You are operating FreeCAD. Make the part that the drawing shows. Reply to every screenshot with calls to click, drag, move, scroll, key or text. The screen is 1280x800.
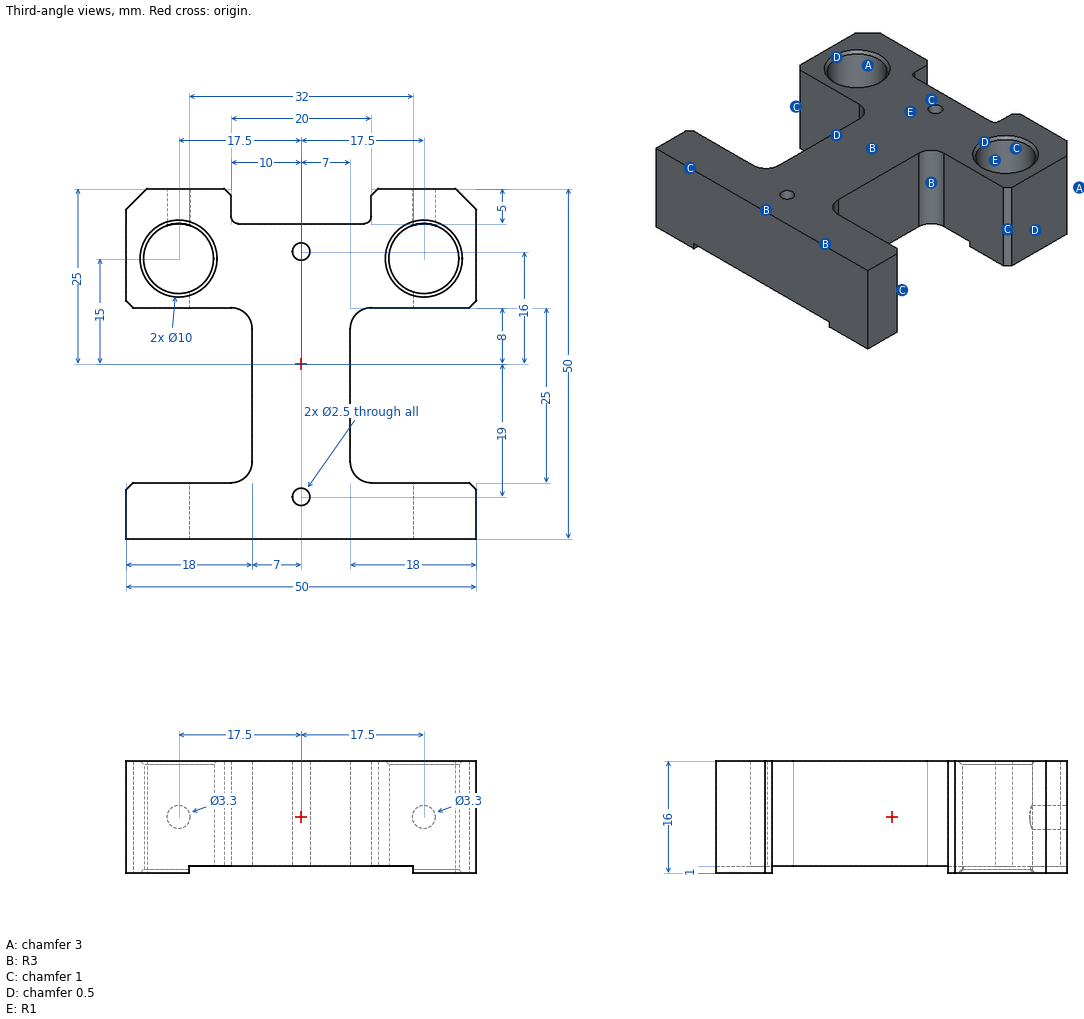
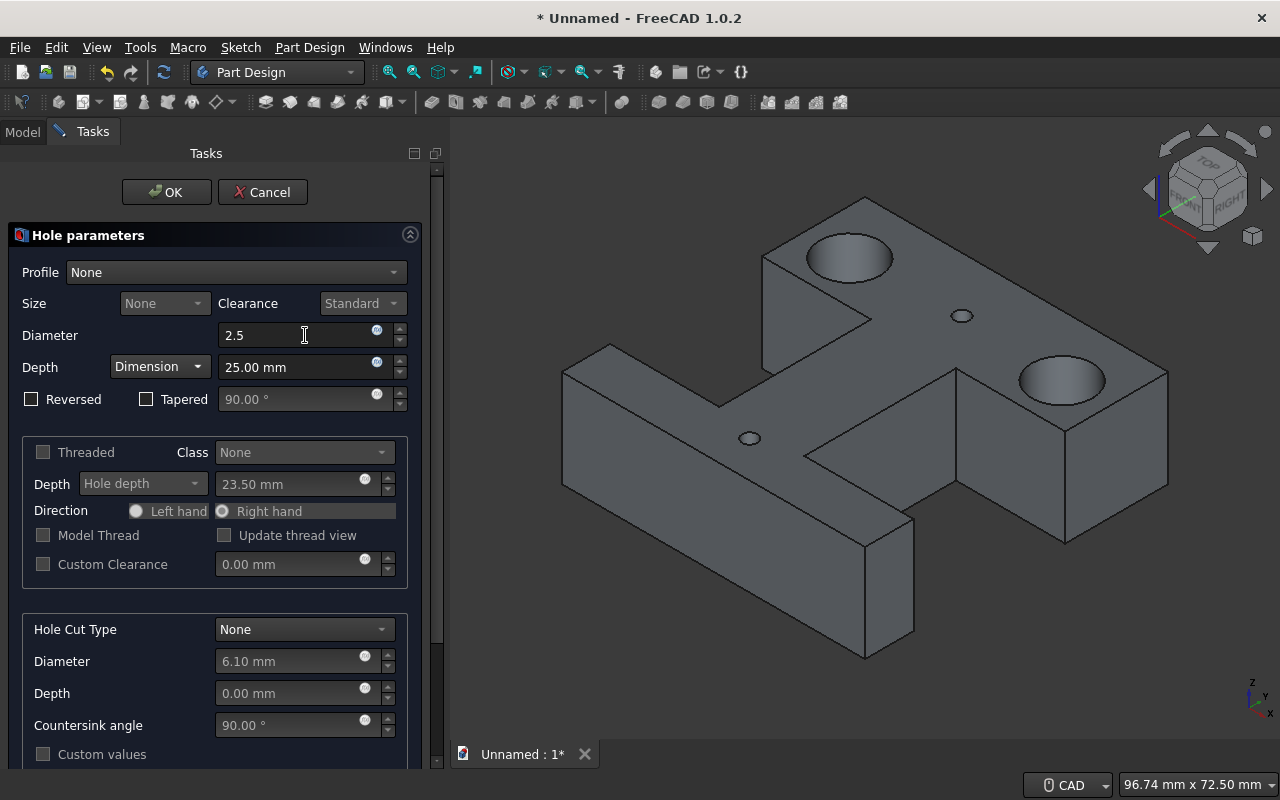
click(161, 366)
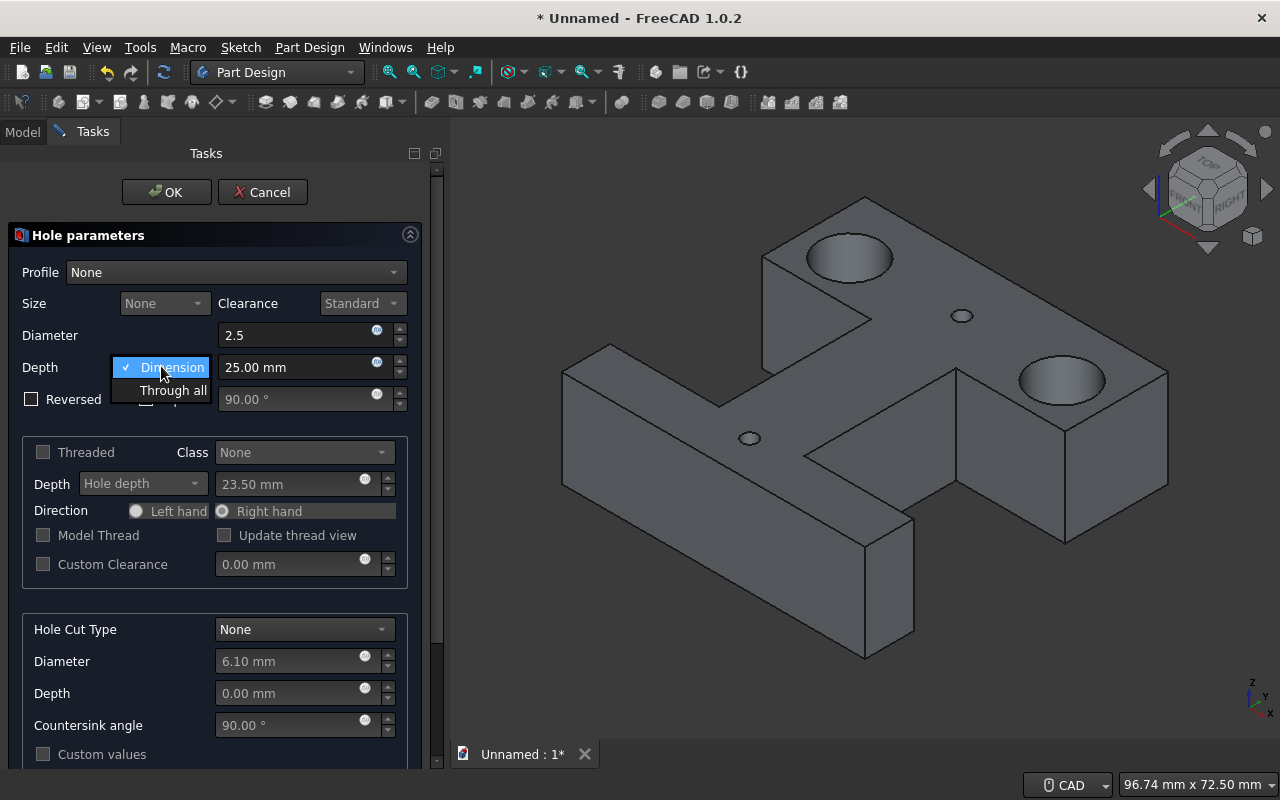
click(160, 390)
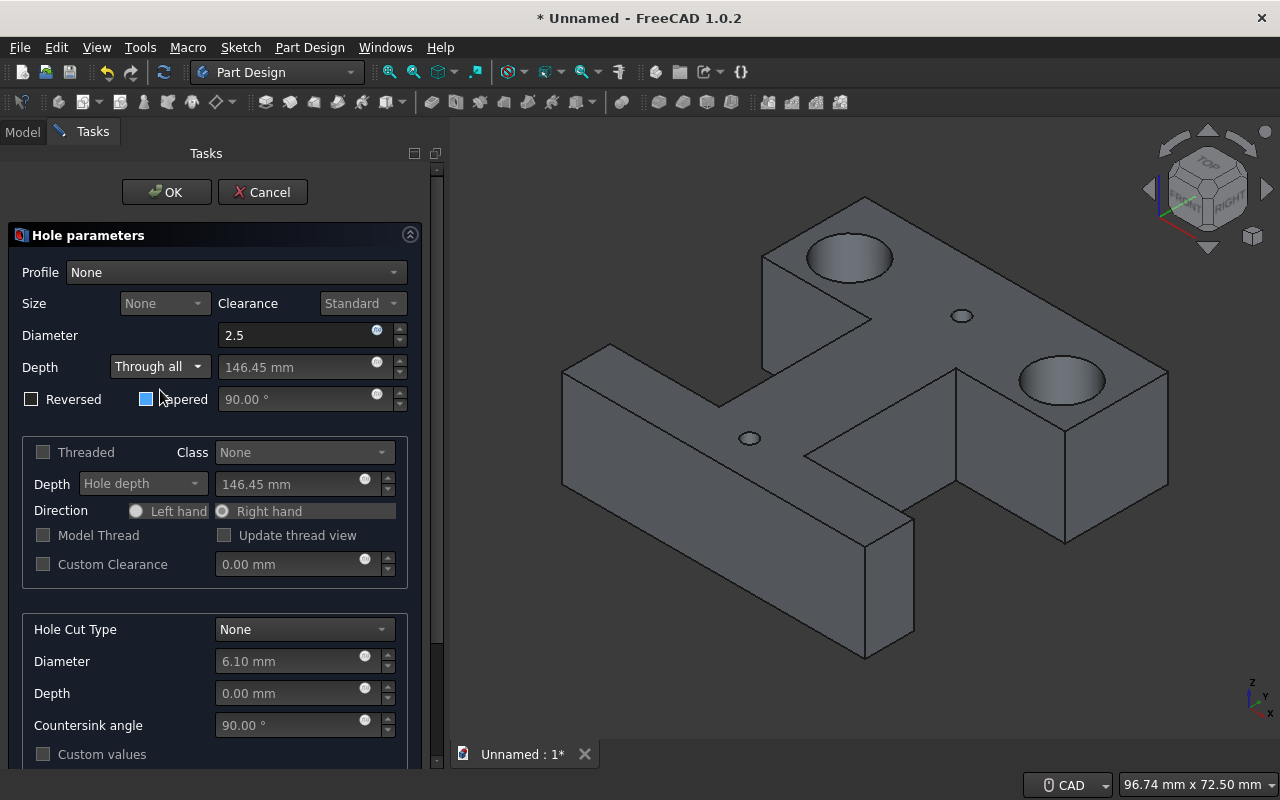
click(167, 192)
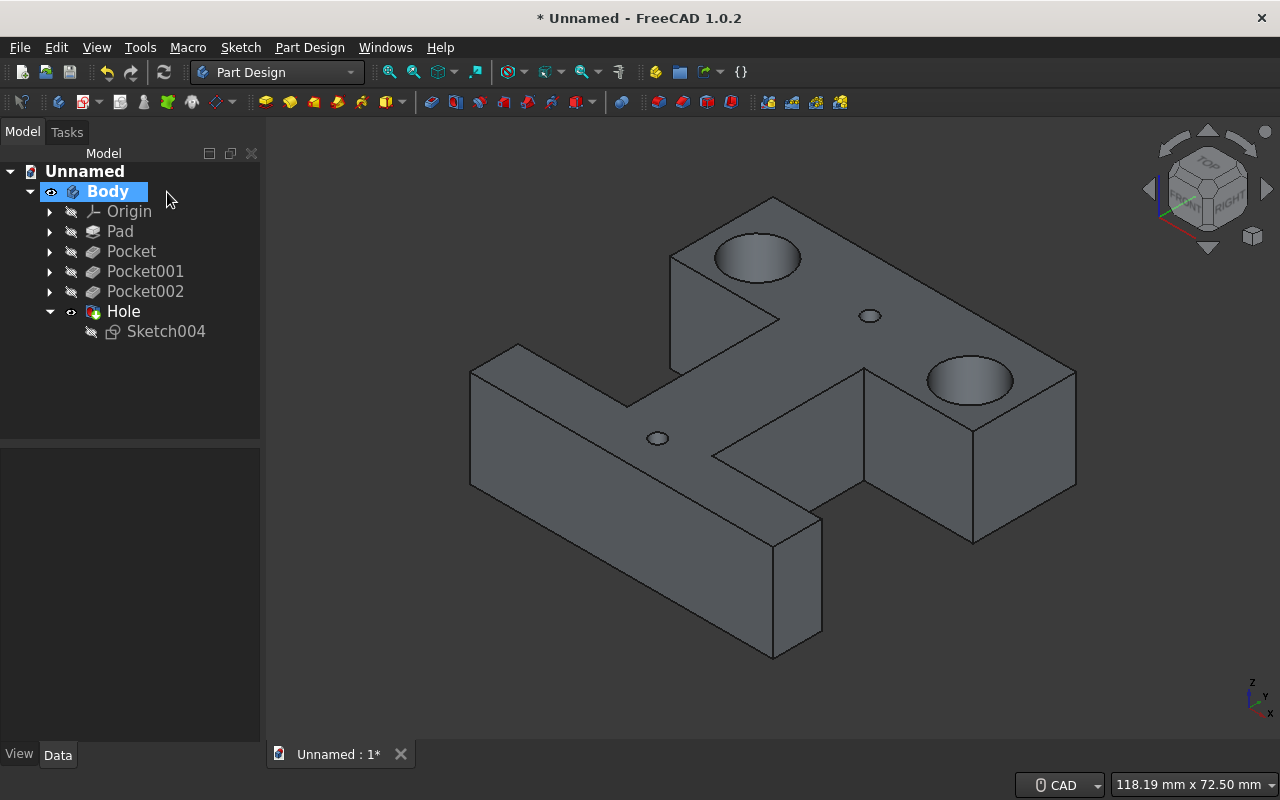
key(5)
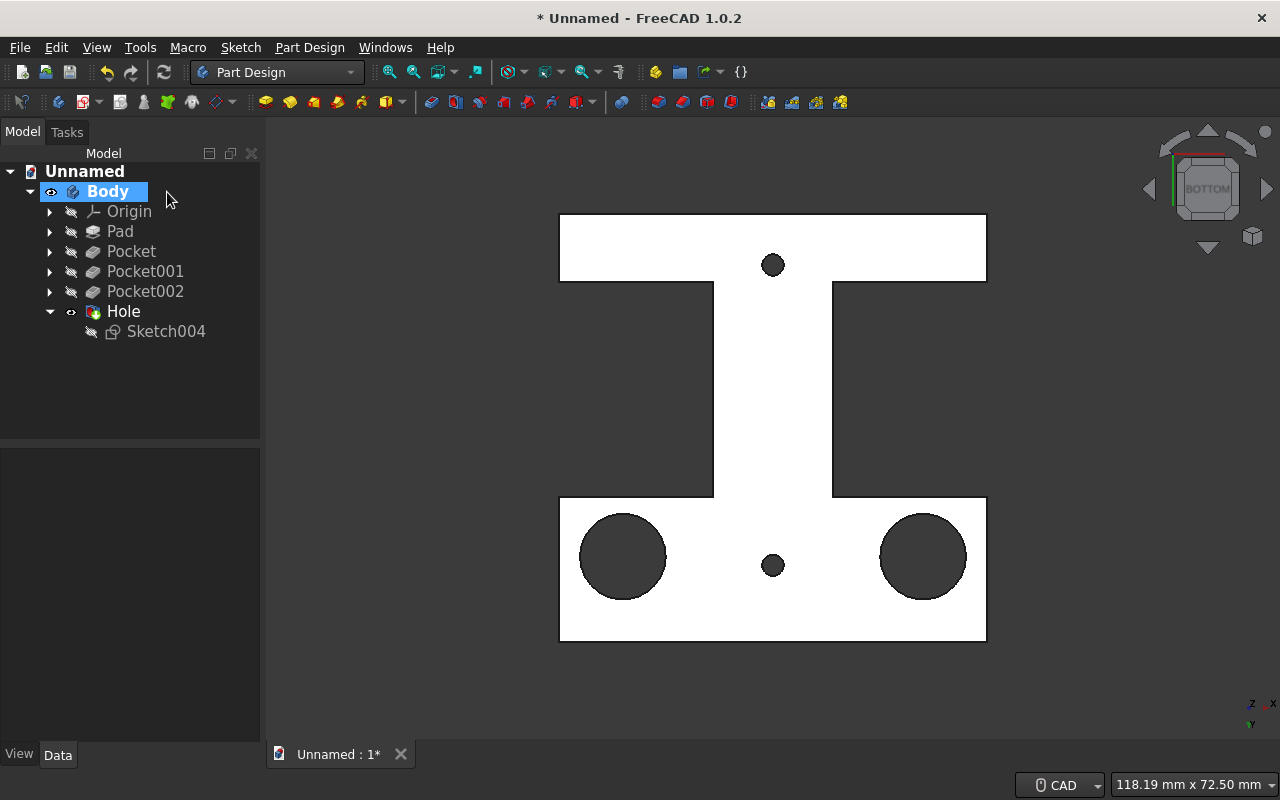
click(773, 488)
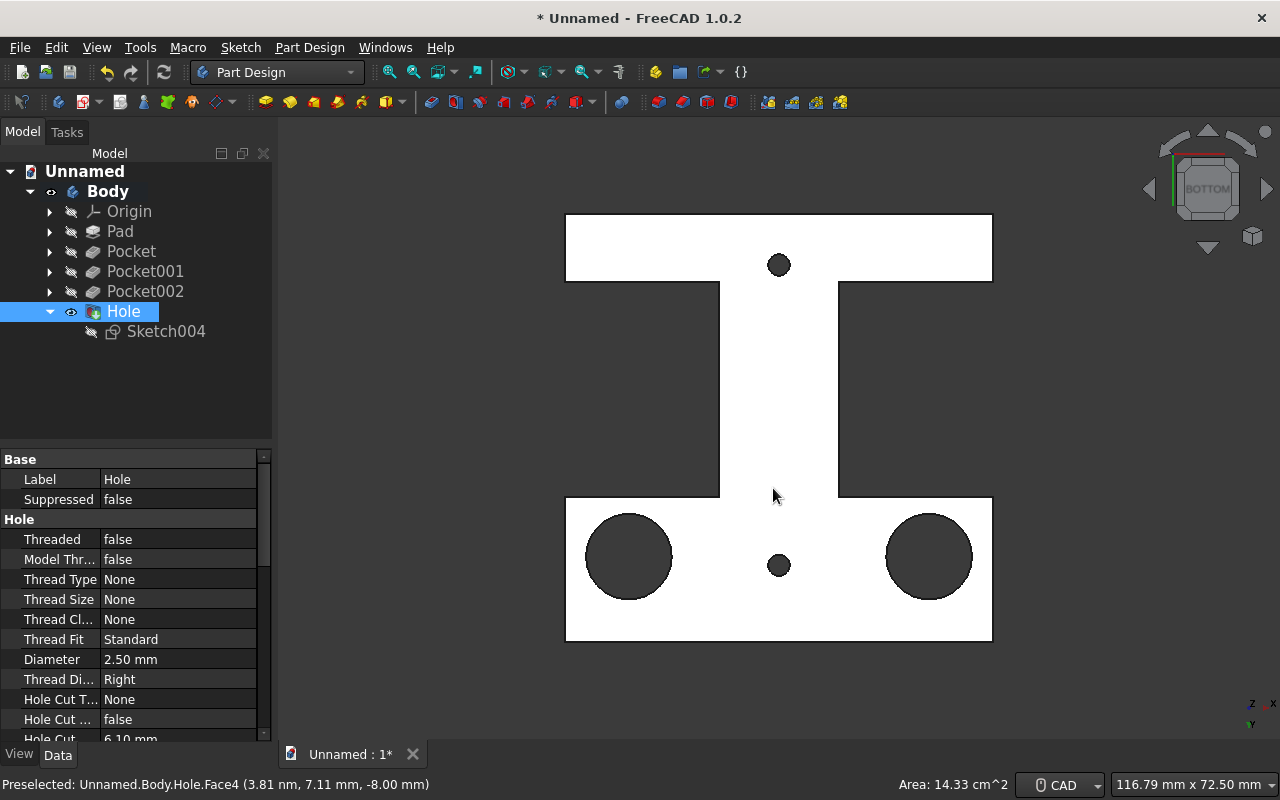
click(84, 102)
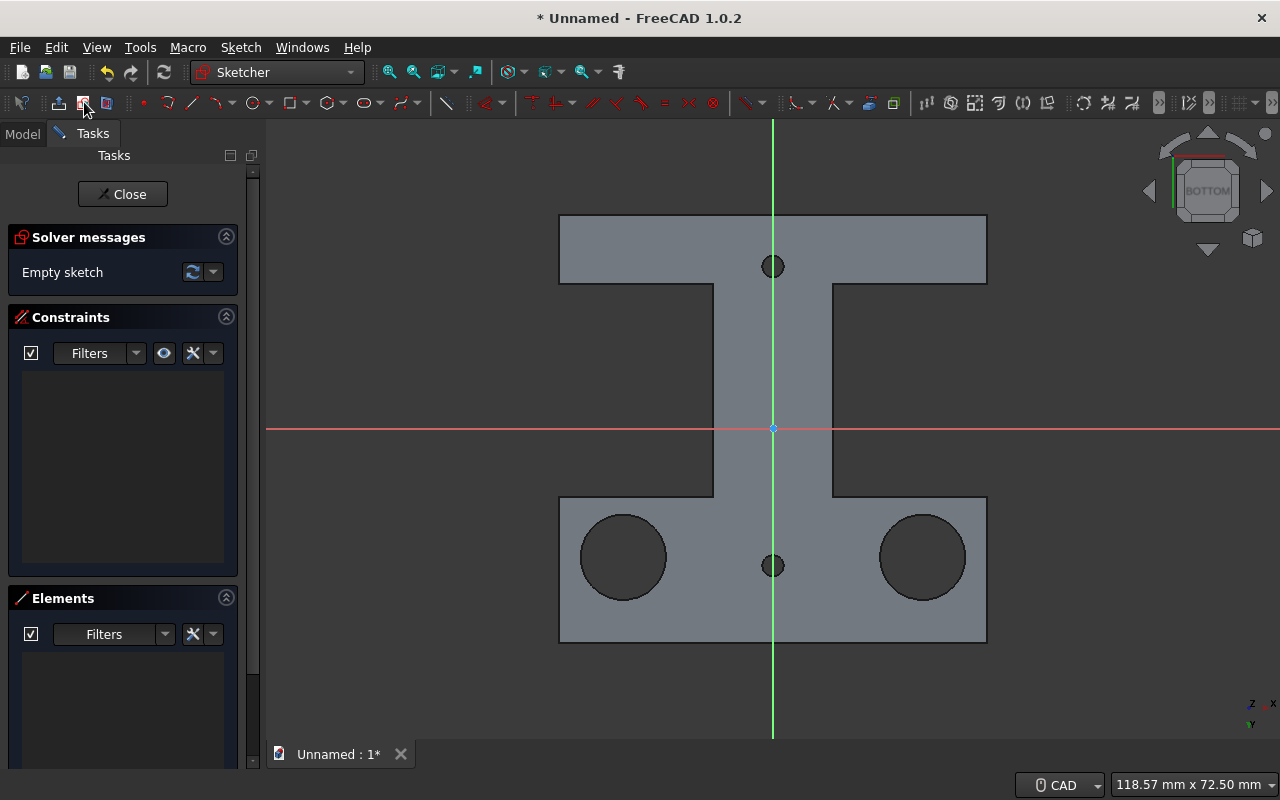
key(g)
key(v)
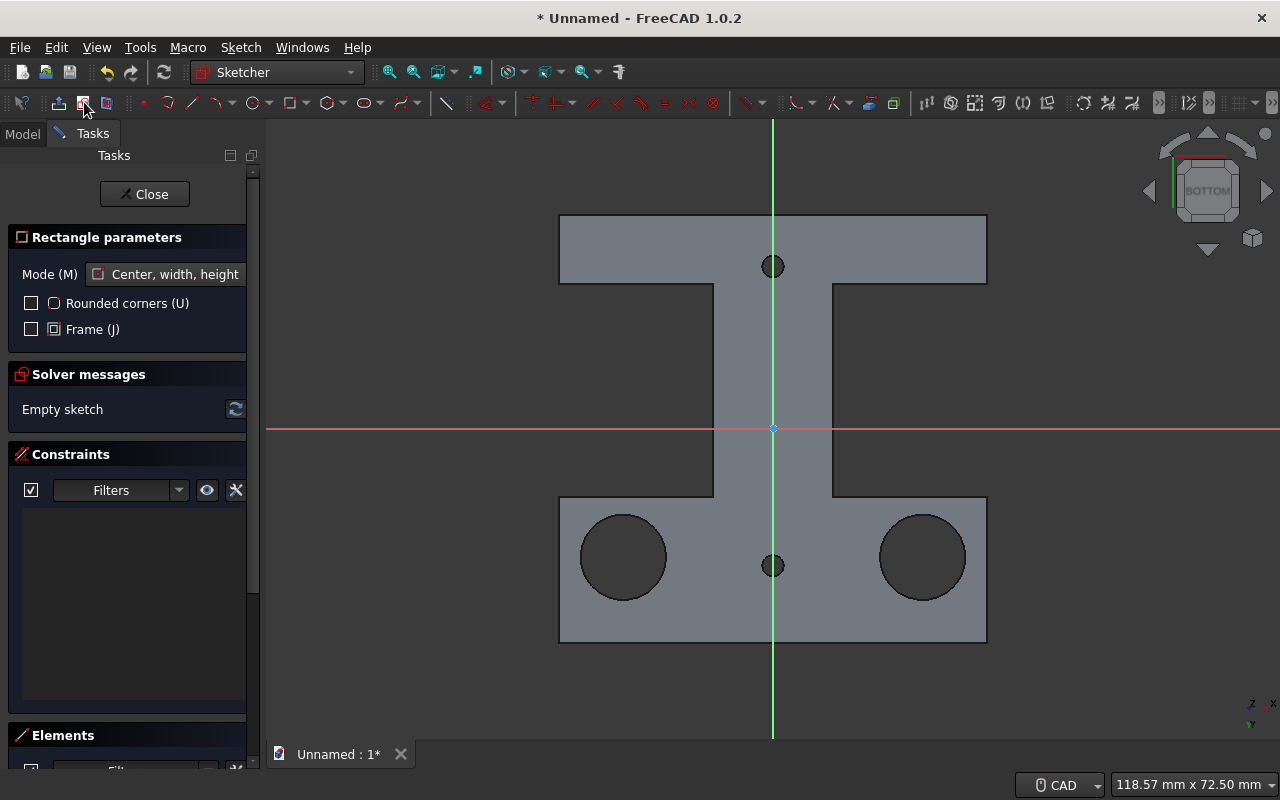
click(773, 429)
move(910, 215)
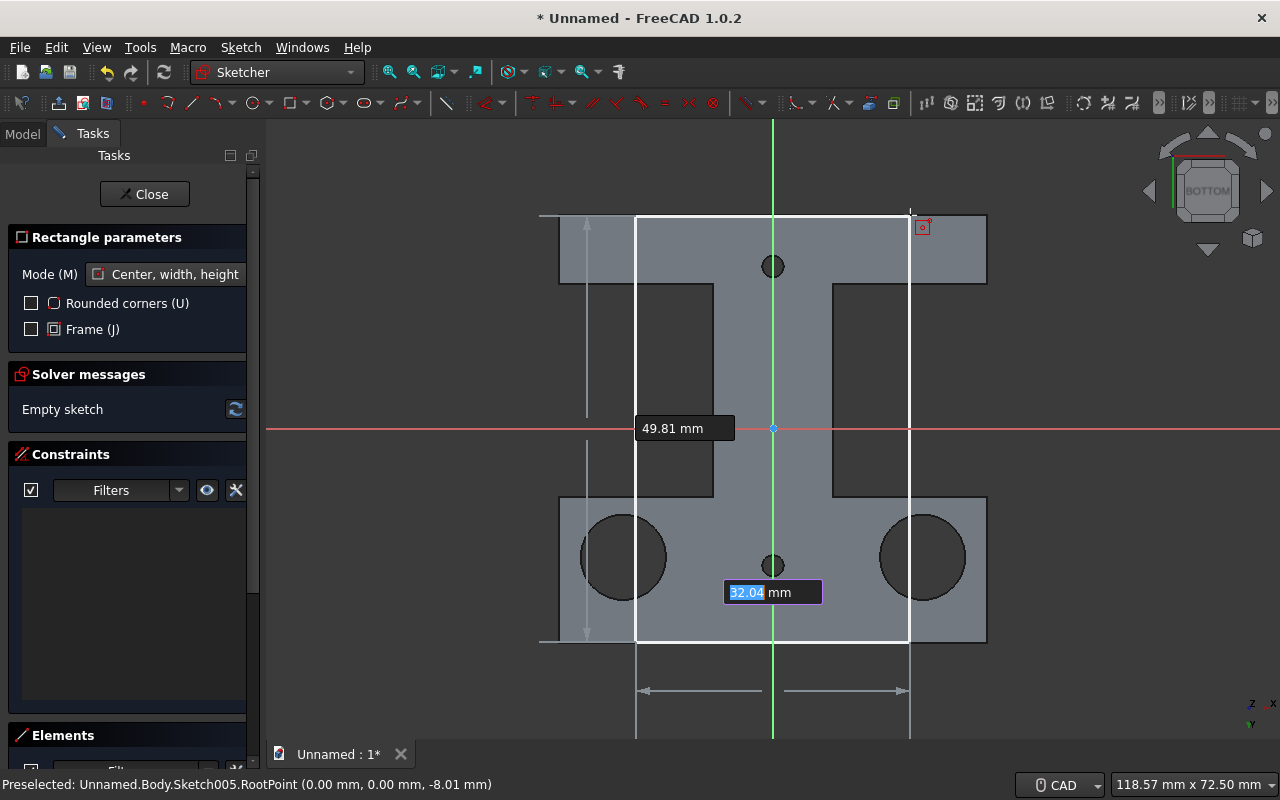
text(32)
key(Tab)
text(50)
key(Return)
key(Escape)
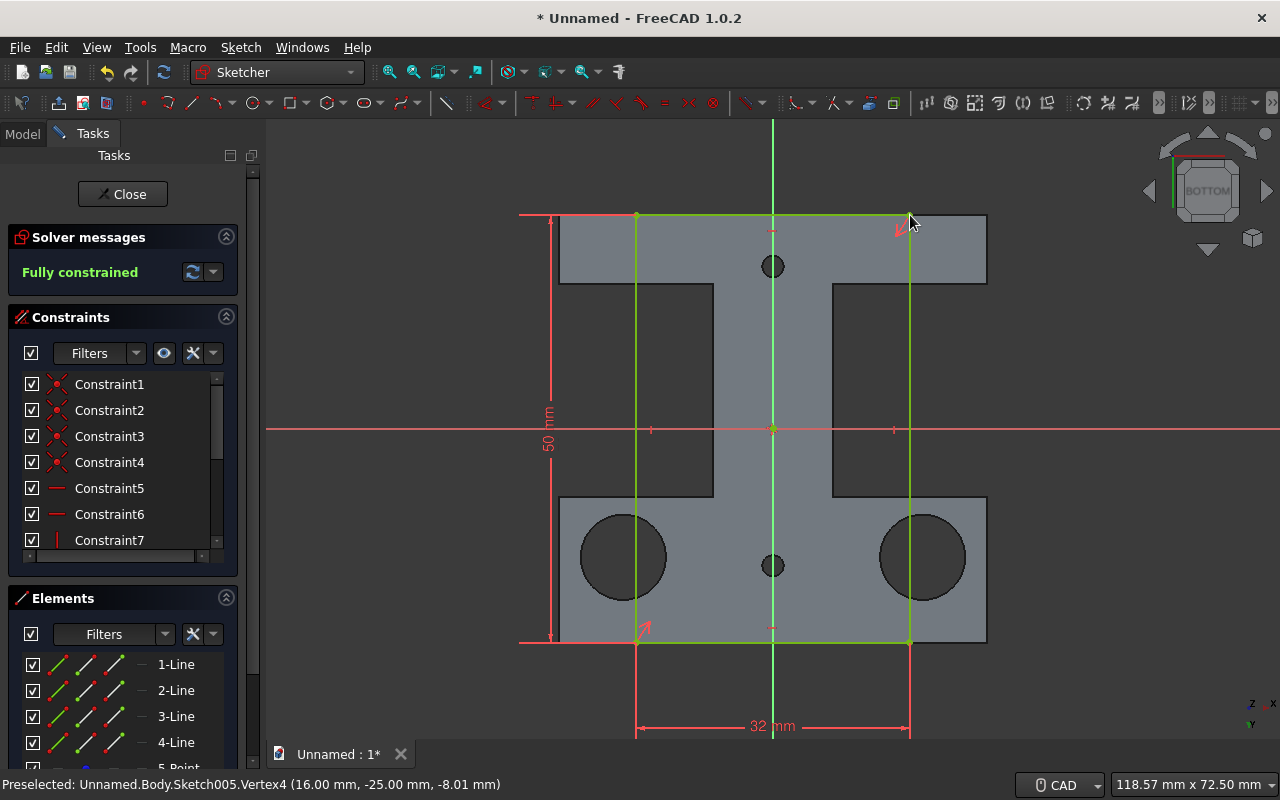
click(123, 194)